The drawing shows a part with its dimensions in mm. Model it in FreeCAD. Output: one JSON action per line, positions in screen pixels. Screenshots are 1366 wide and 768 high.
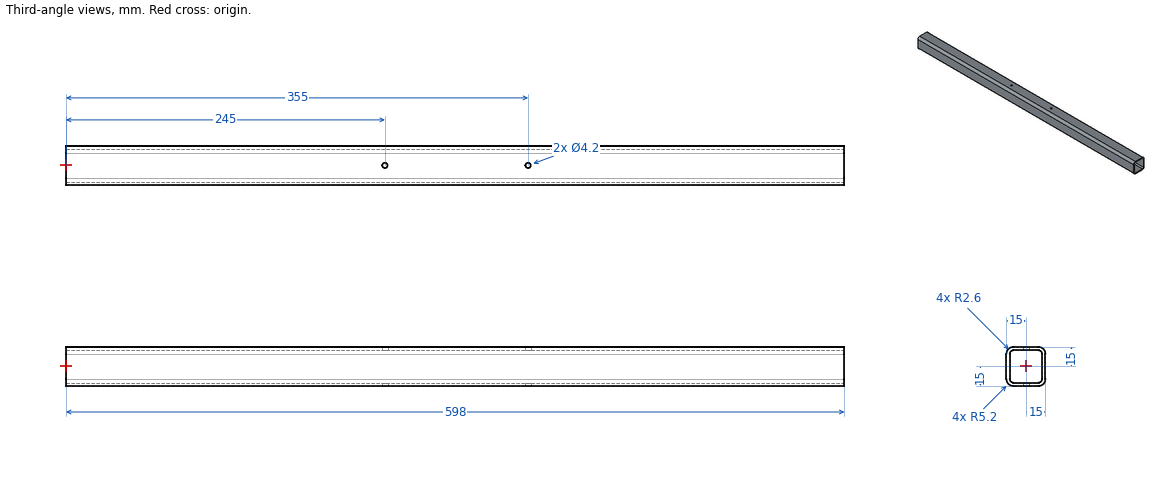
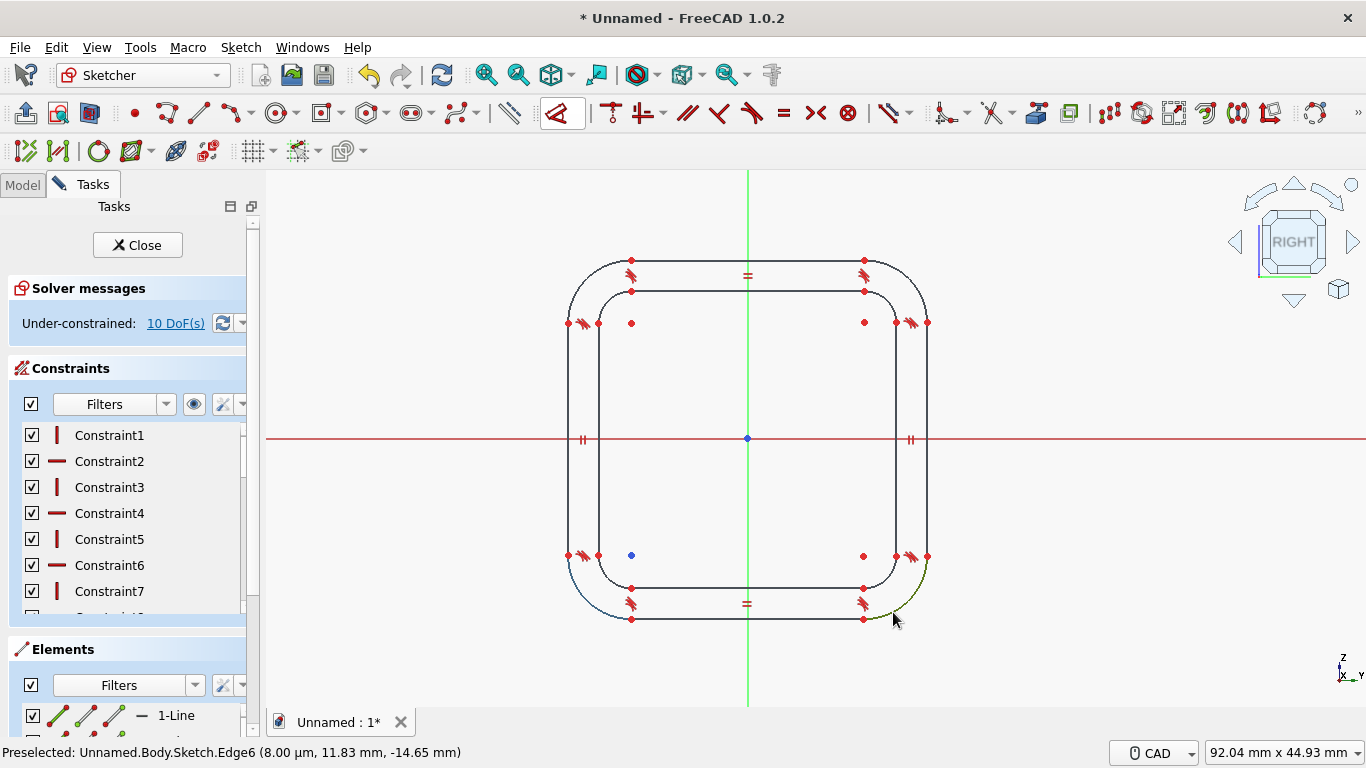
{"action": "left_click", "coordinate": [920, 294]}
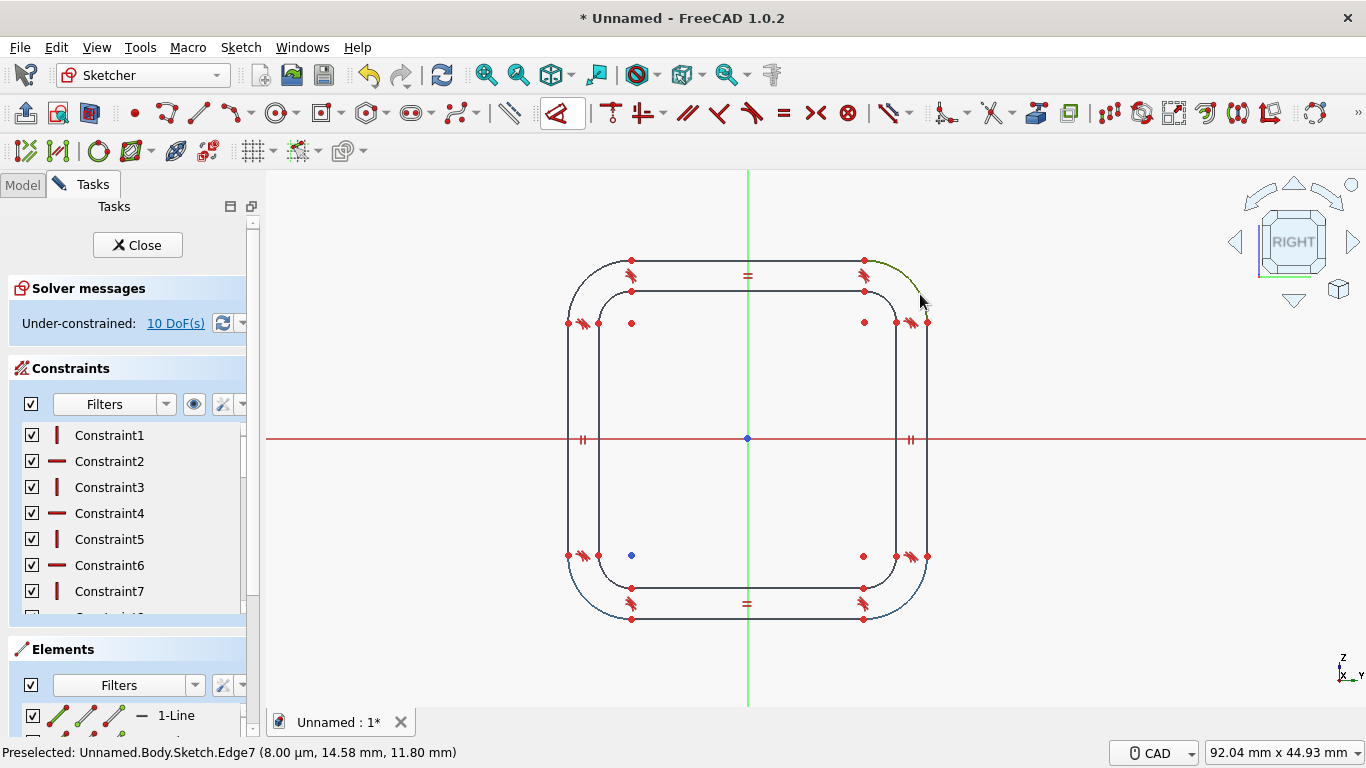
{"action": "left_click", "coordinate": [603, 267]}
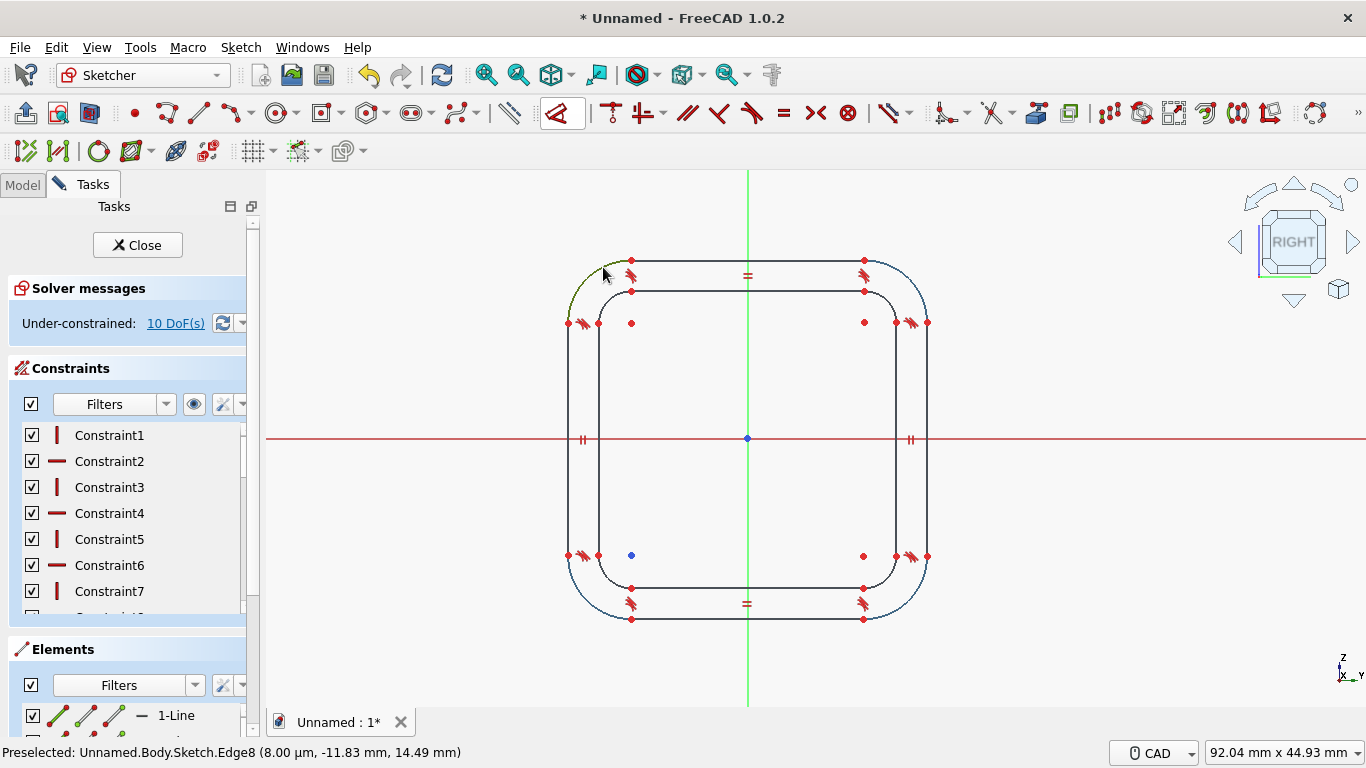
{"action": "key", "text": "e"}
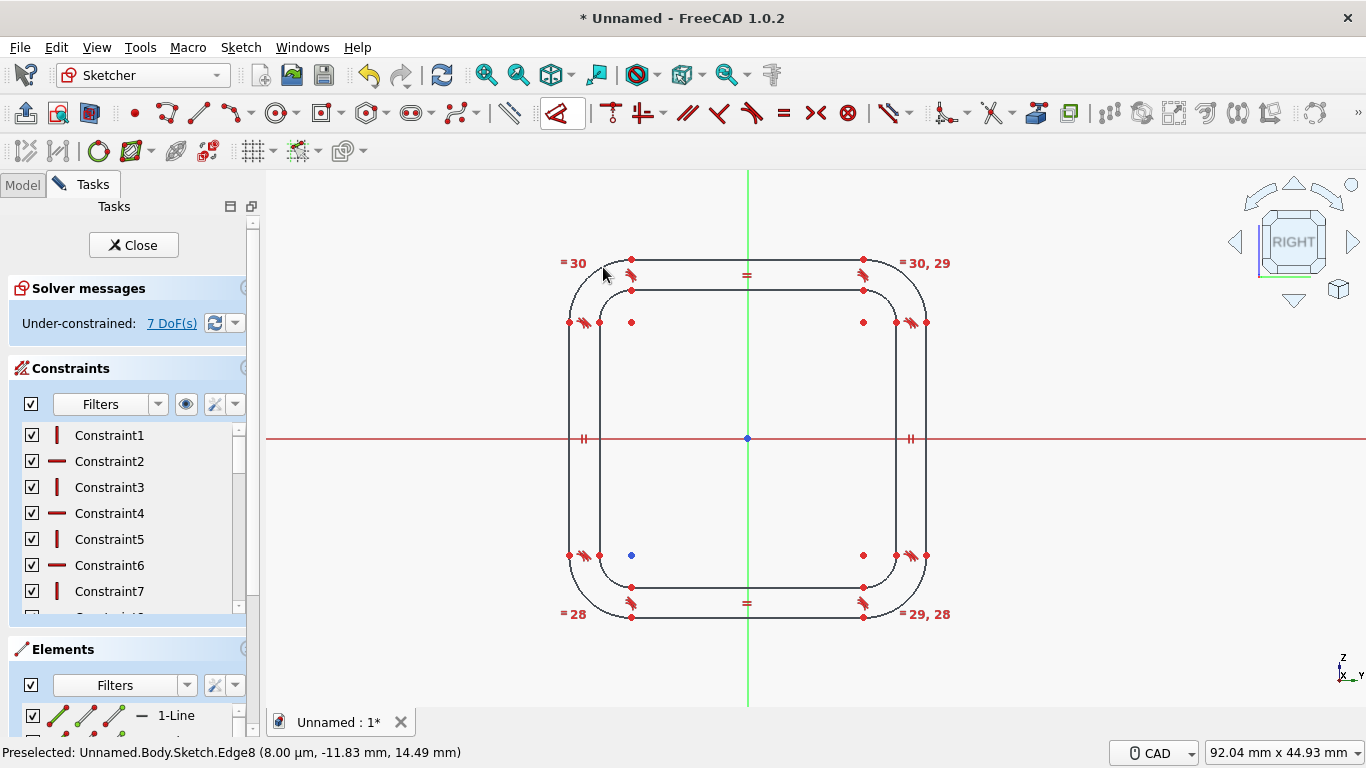
{"action": "left_click", "coordinate": [617, 294]}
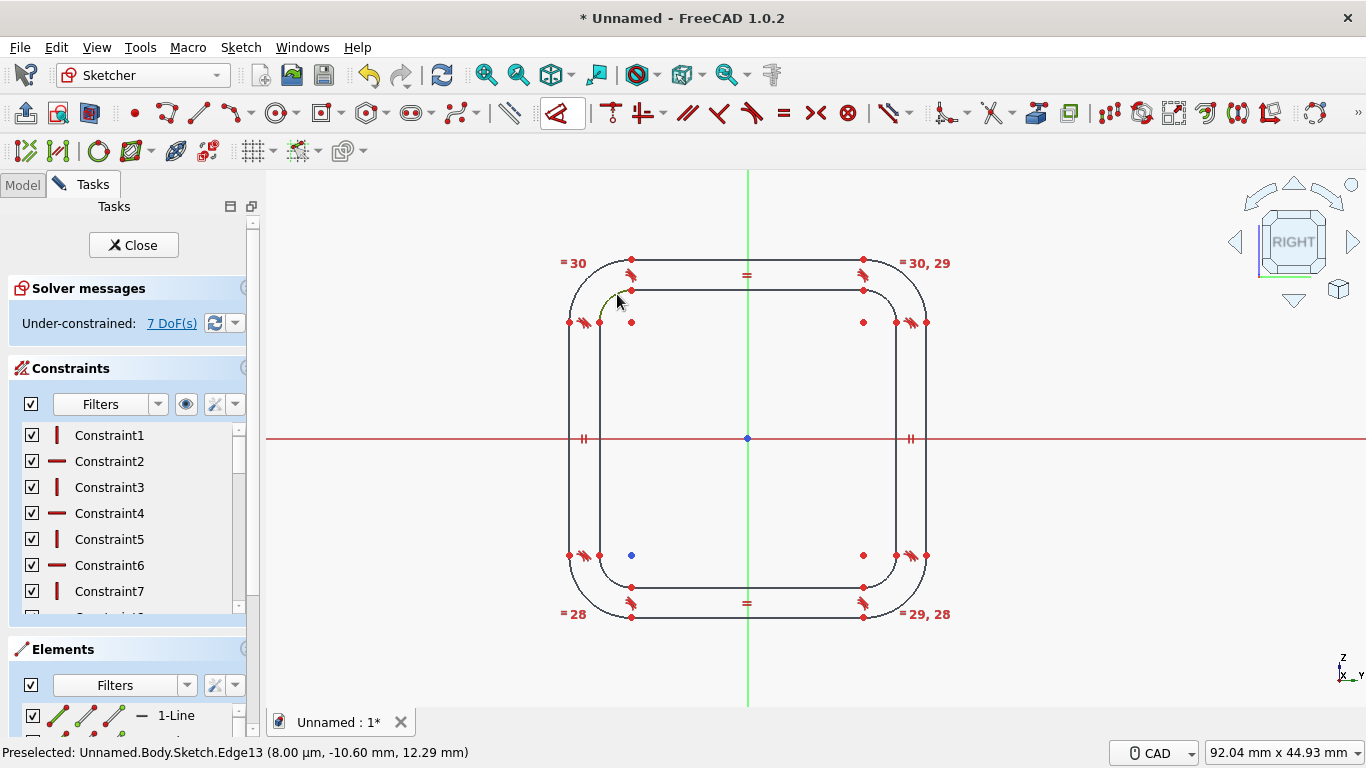
{"action": "left_click", "coordinate": [603, 570]}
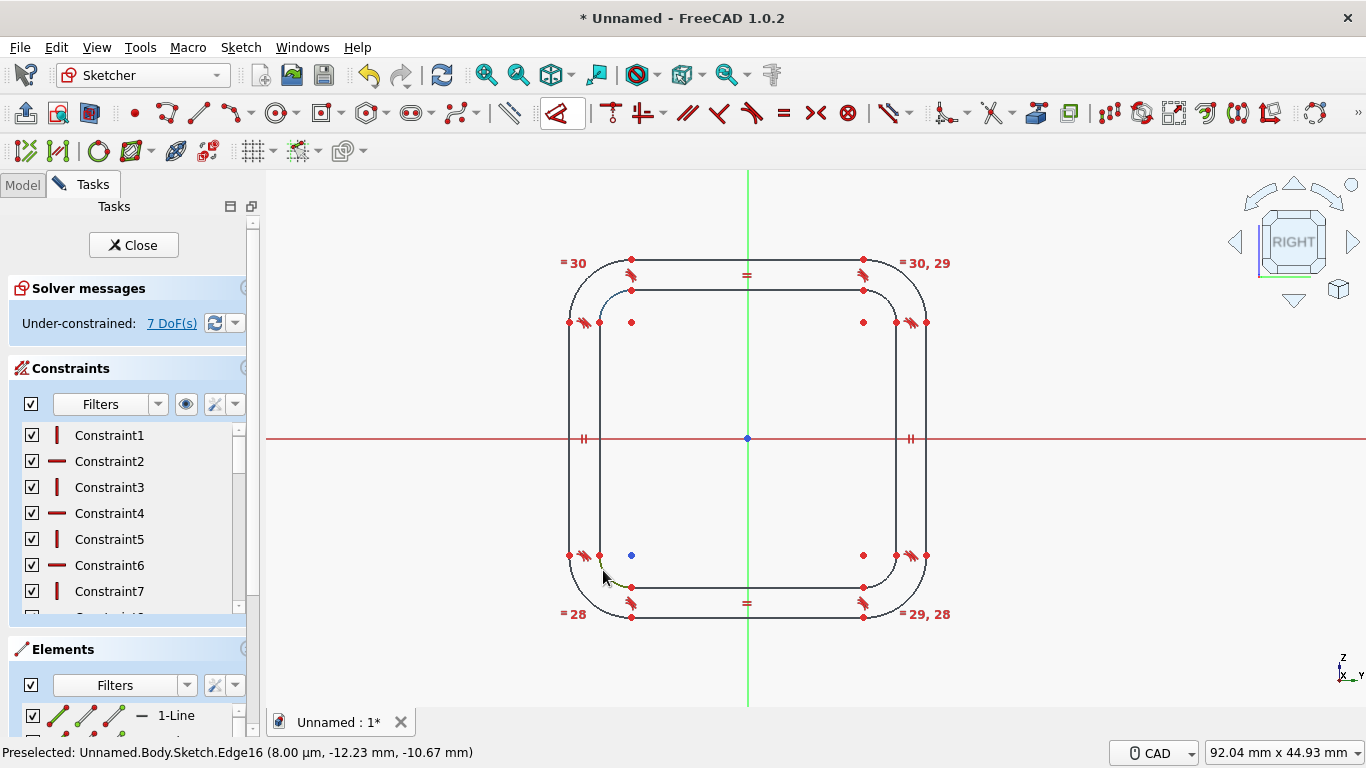
{"action": "left_click", "coordinate": [784, 114]}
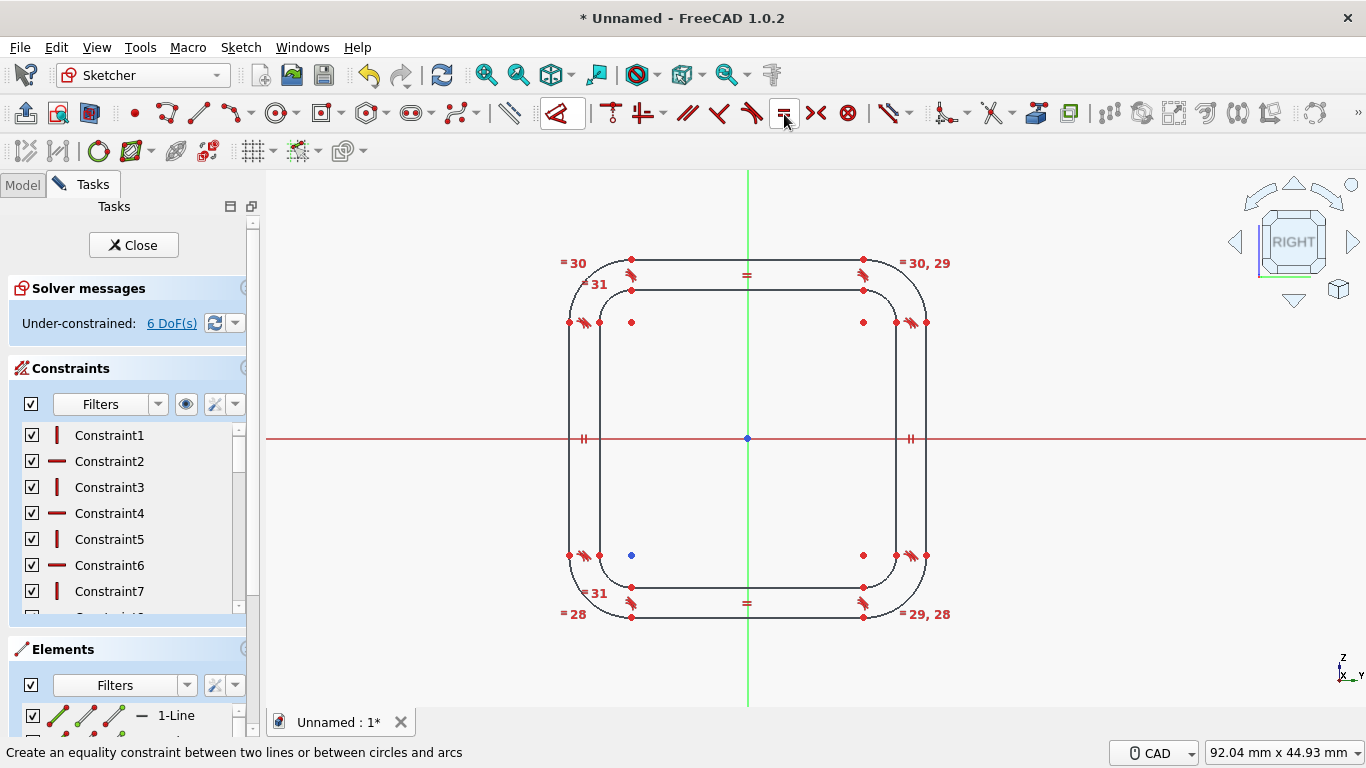
{"action": "key", "text": "d"}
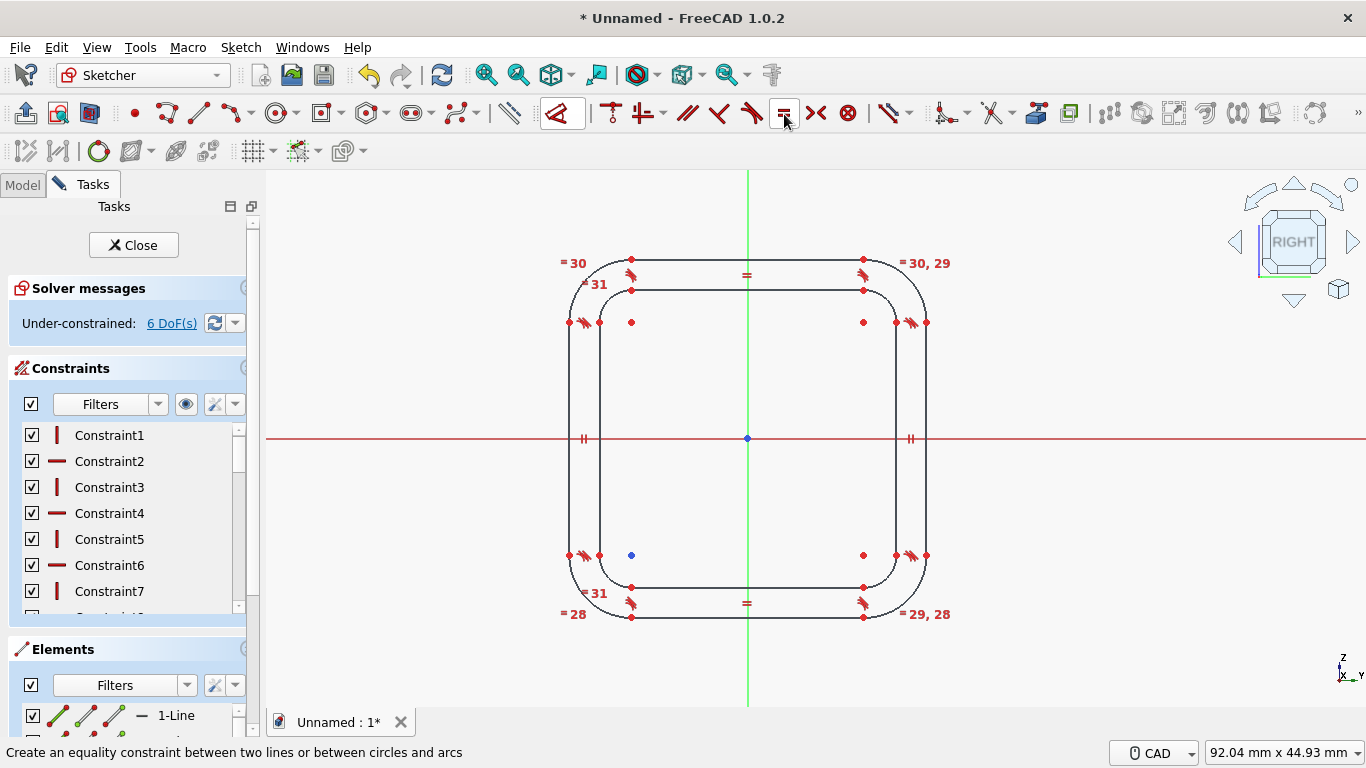
{"action": "left_click", "coordinate": [576, 584]}
{"action": "left_click", "coordinate": [548, 599]}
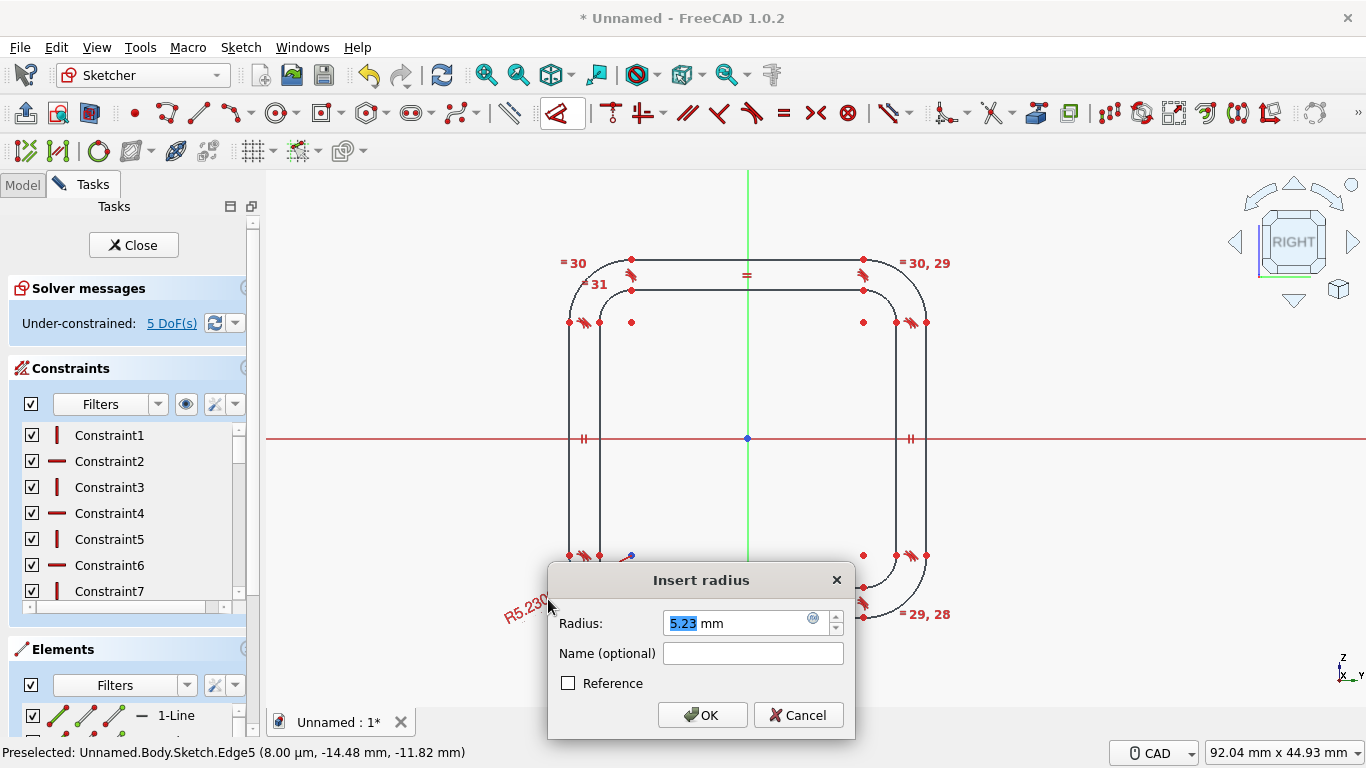
{"action": "type", "text": "5.2"}
{"action": "key", "text": "Return"}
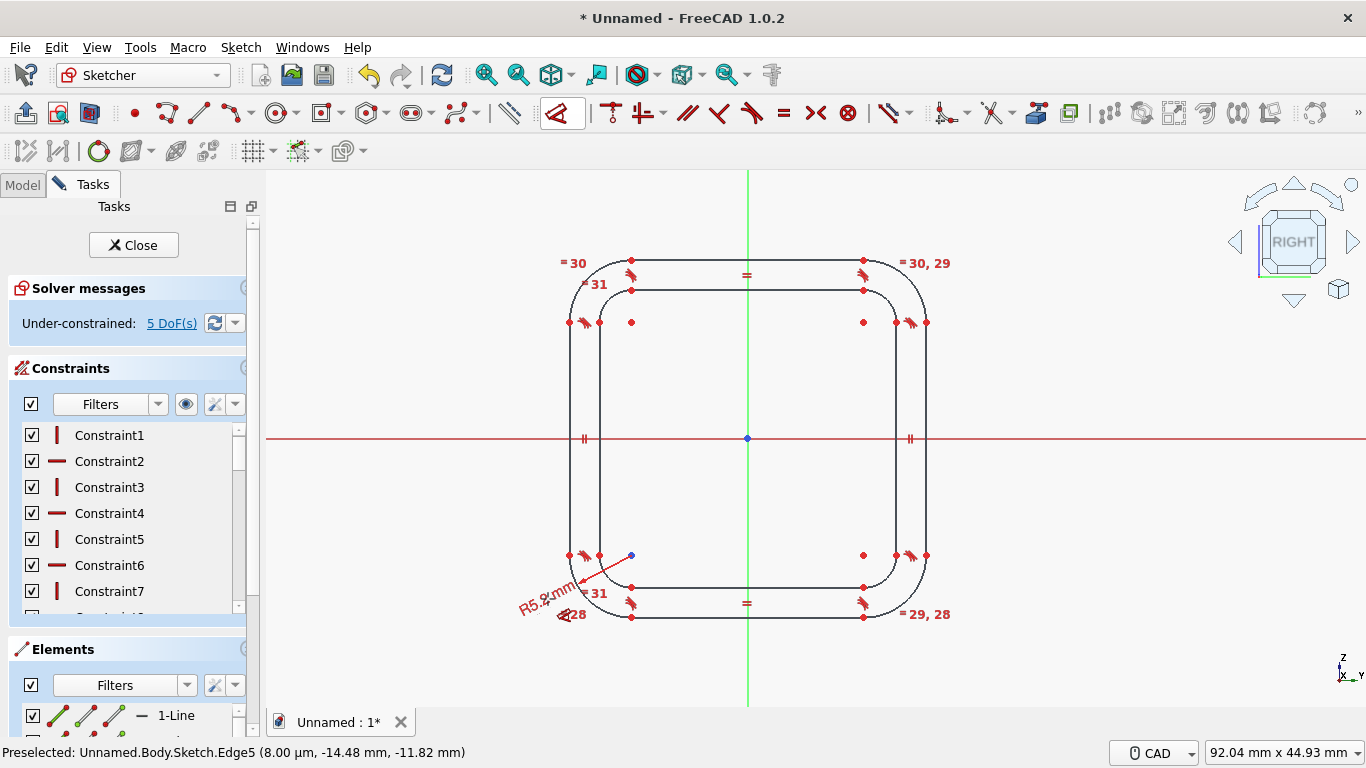
{"action": "scroll", "coordinate": [617, 294], "scroll_direction": "up", "scroll_amount": 2}